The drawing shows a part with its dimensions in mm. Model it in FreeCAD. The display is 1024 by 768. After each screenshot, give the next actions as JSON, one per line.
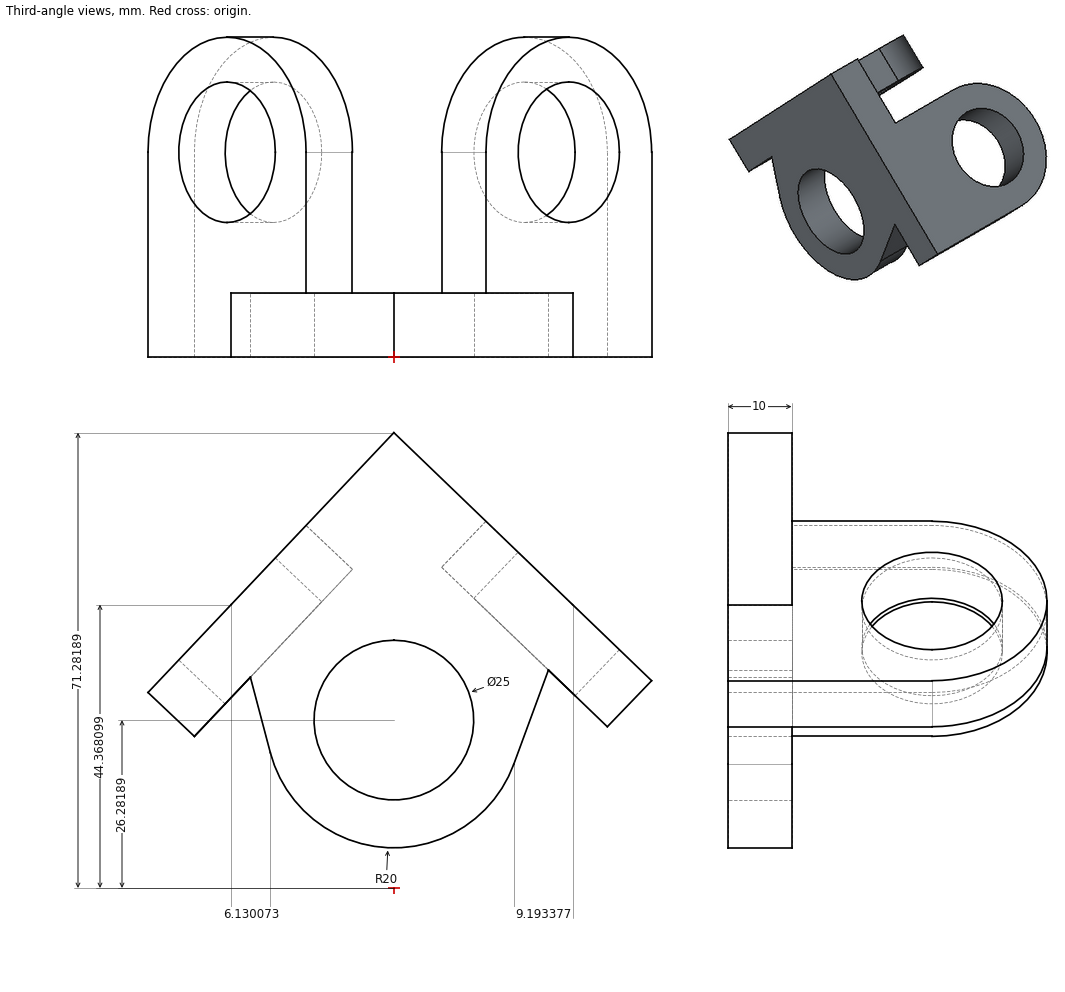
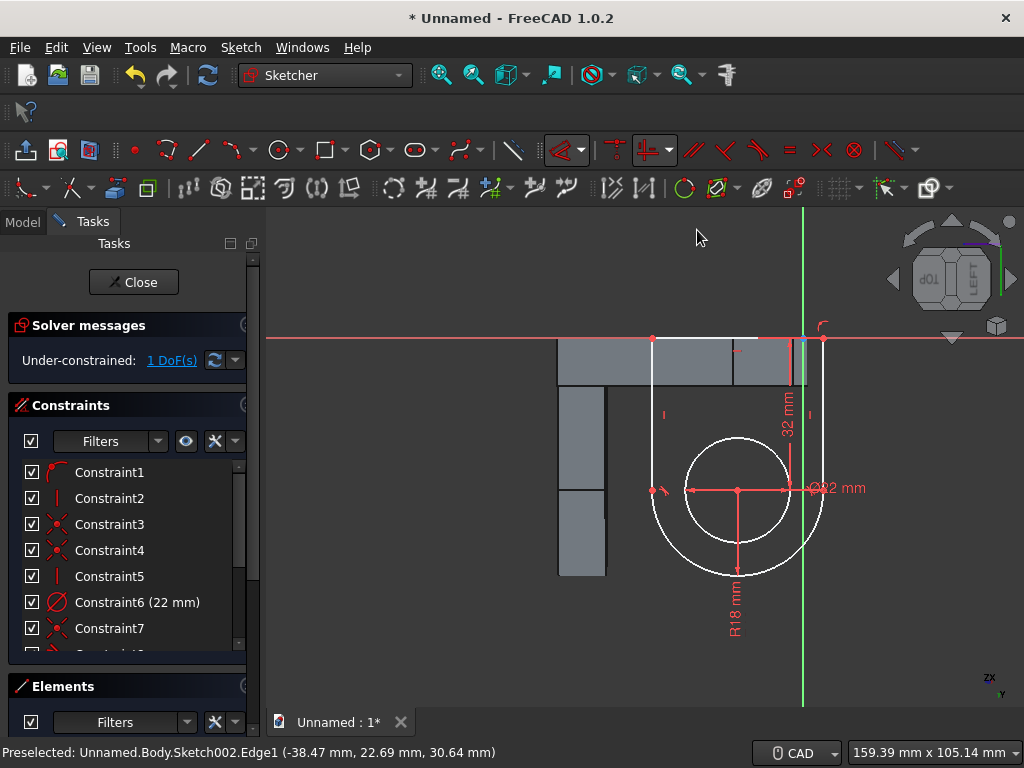
{"action": "scroll", "coordinate": [823, 490], "scroll_direction": "up", "scroll_amount": 4}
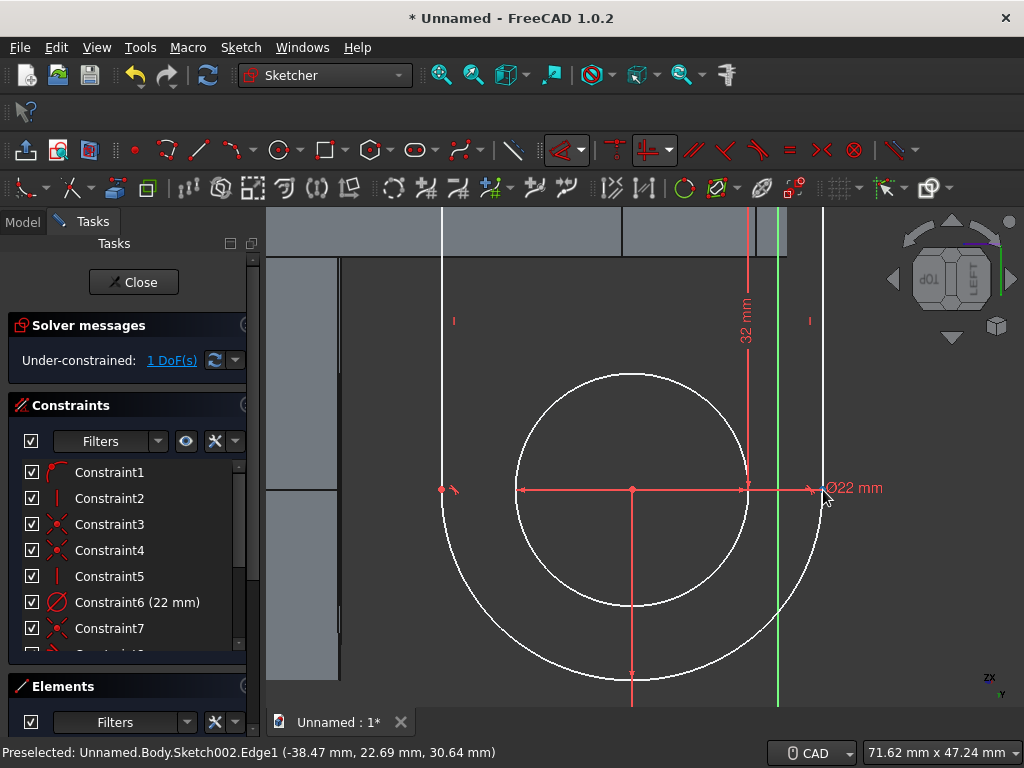
{"action": "left_click", "coordinate": [823, 490]}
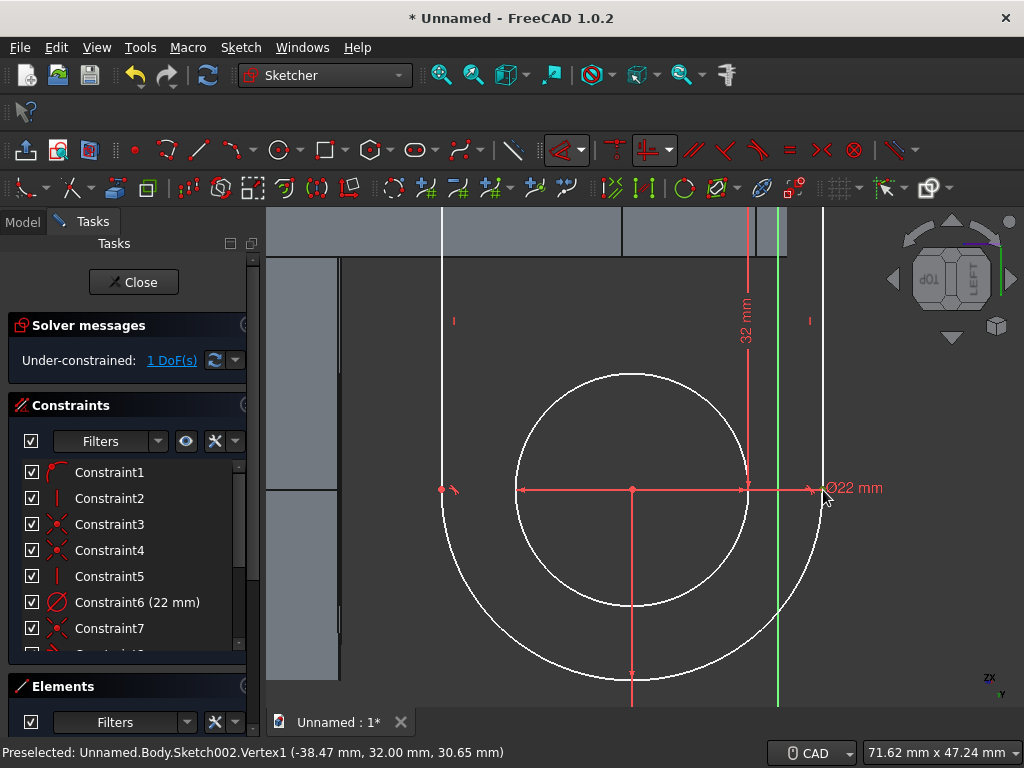
{"action": "key", "text": "l"}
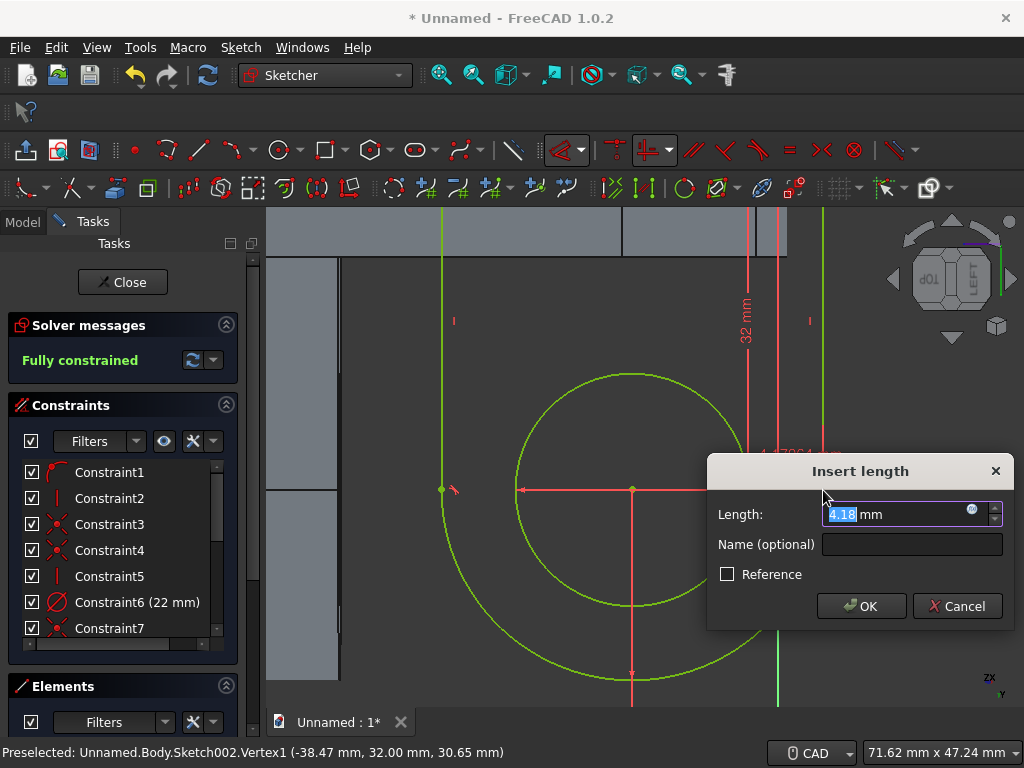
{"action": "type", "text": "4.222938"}
{"action": "key", "text": "Return"}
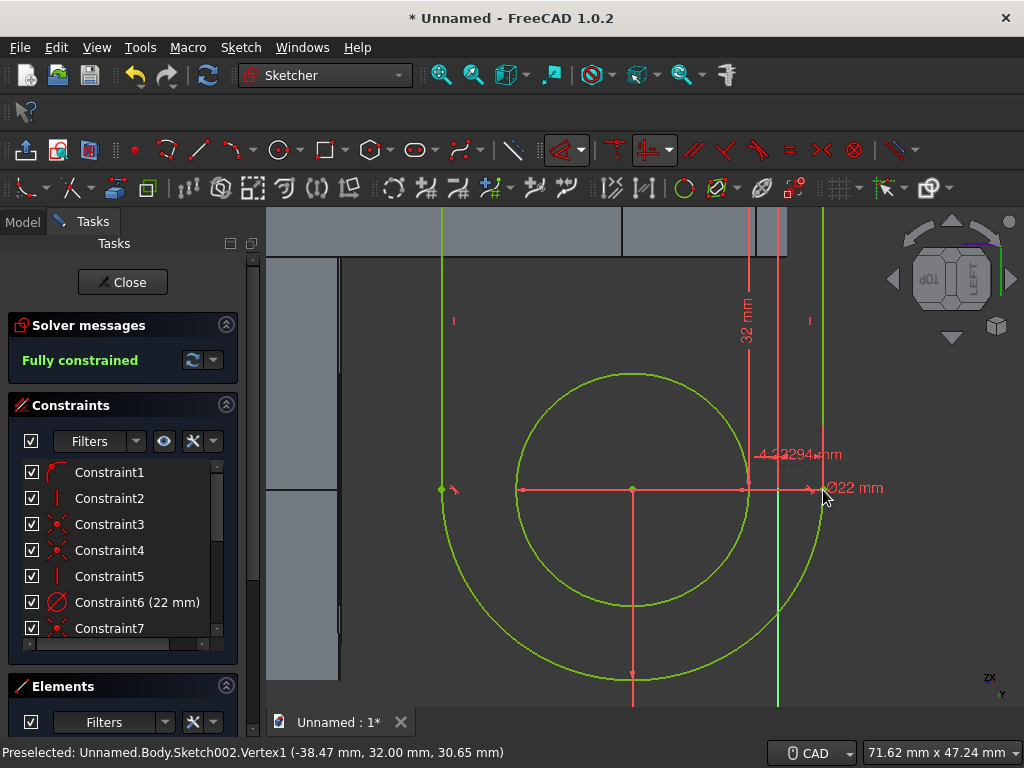
{"action": "left_click", "coordinate": [123, 282]}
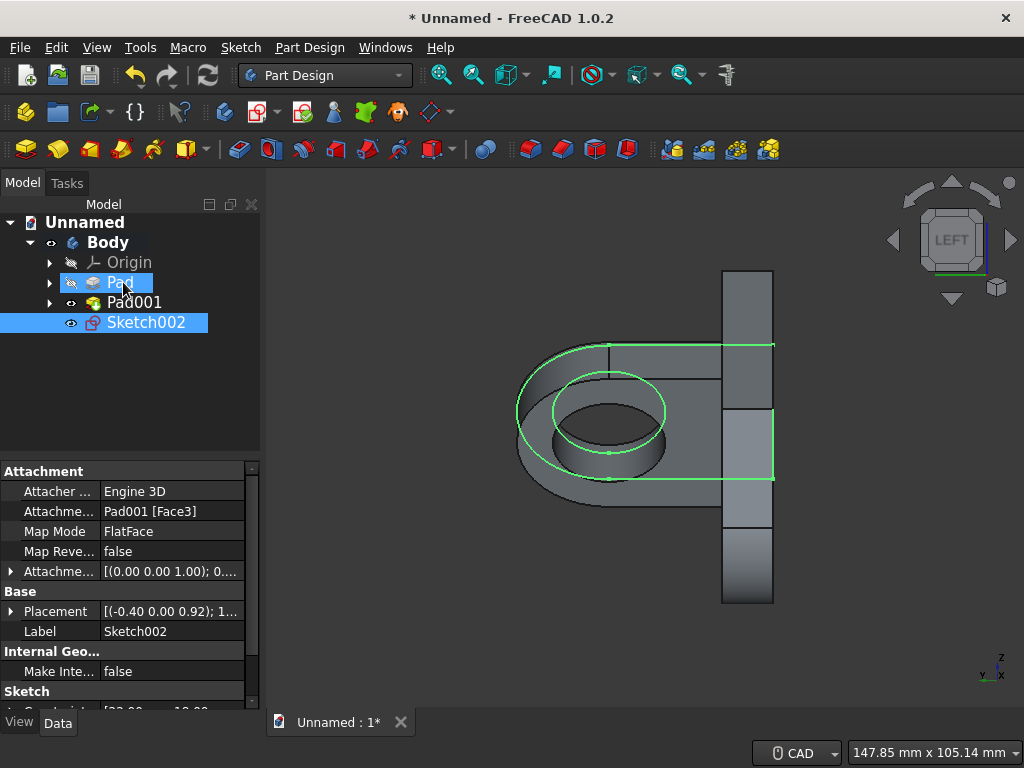
{"action": "left_click", "coordinate": [26, 150]}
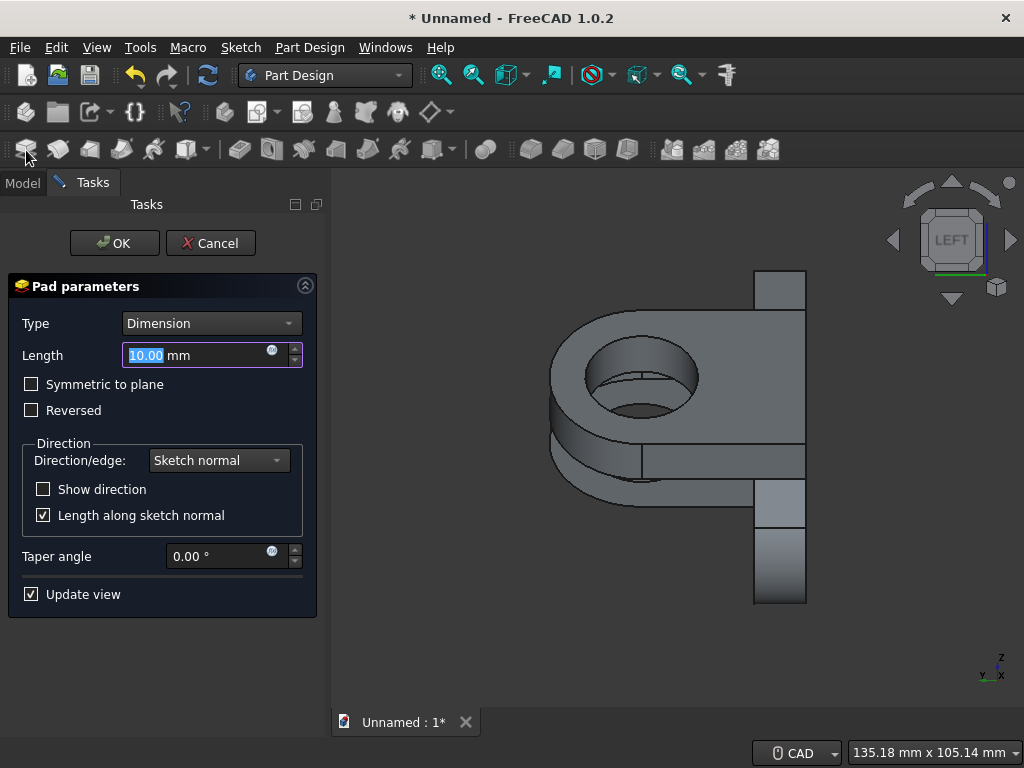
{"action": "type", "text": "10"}
{"action": "key", "text": "Tab"}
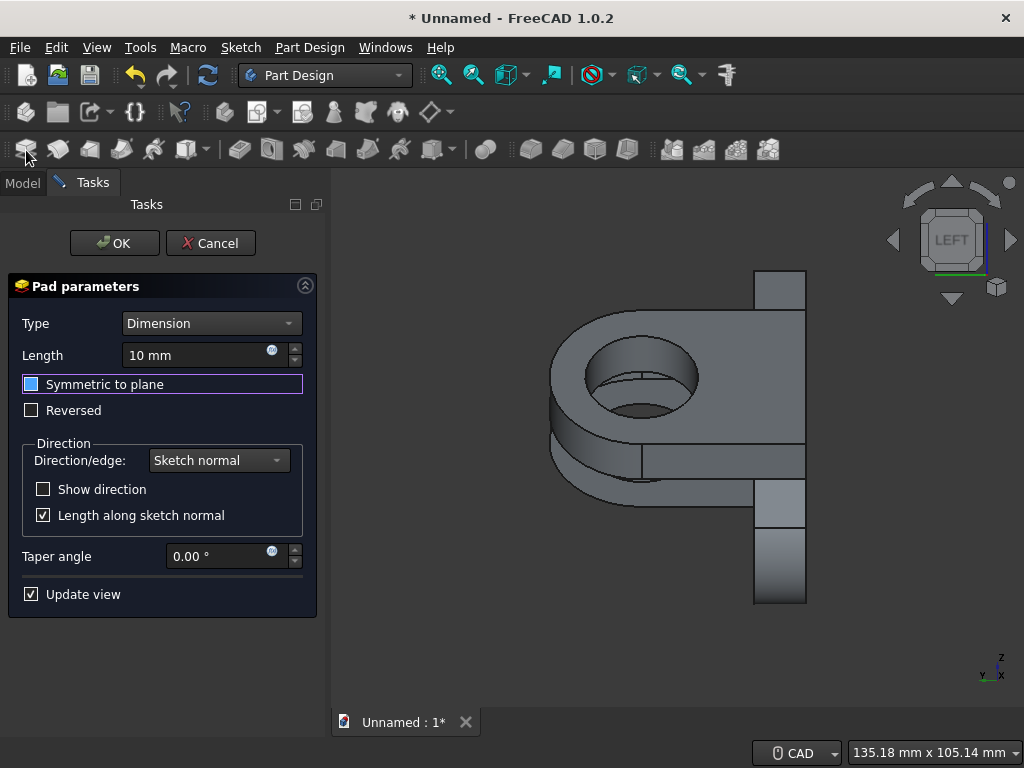
{"action": "left_click", "coordinate": [30, 410]}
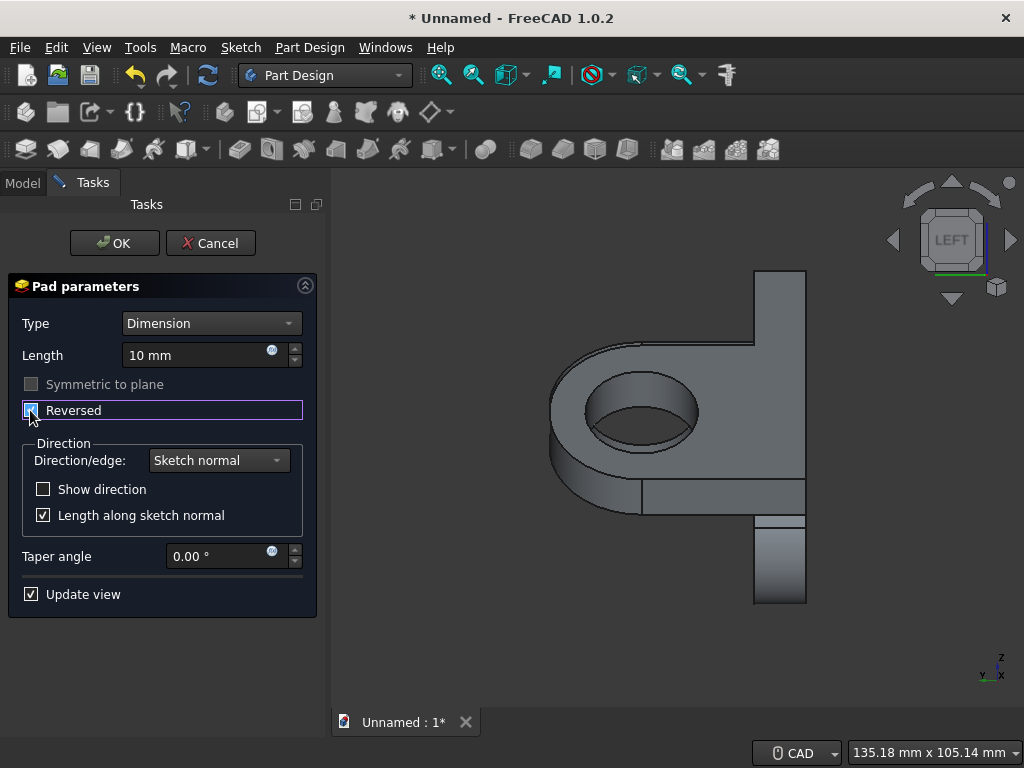
{"action": "left_click", "coordinate": [115, 243]}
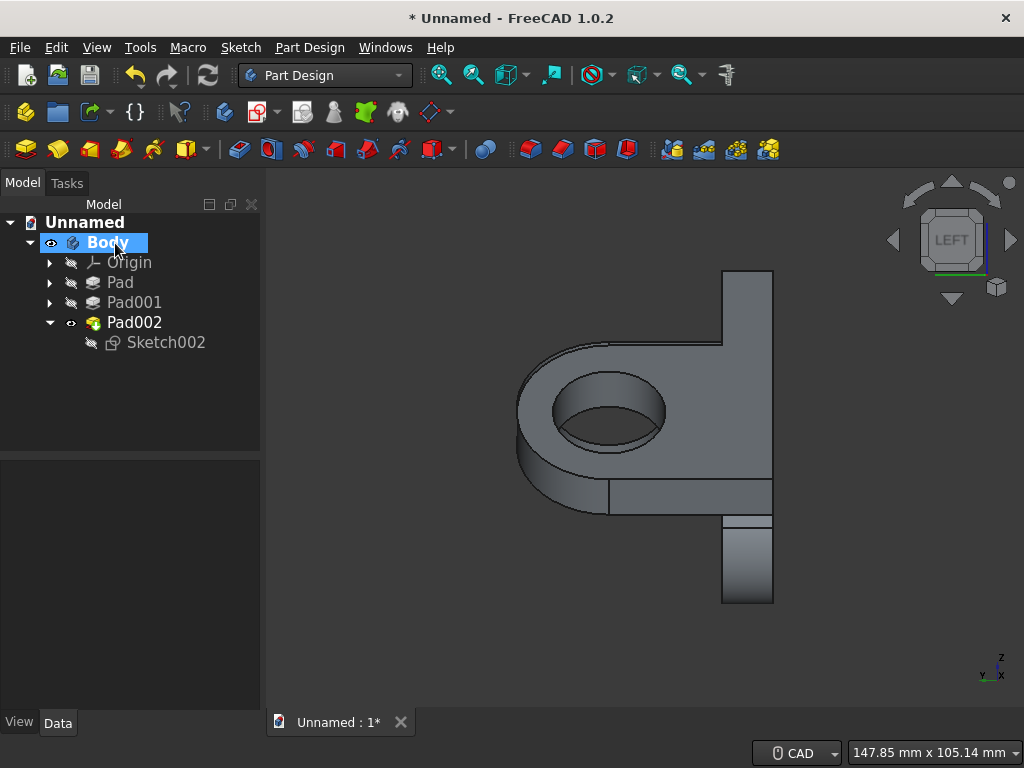
{"action": "key", "text": "0"}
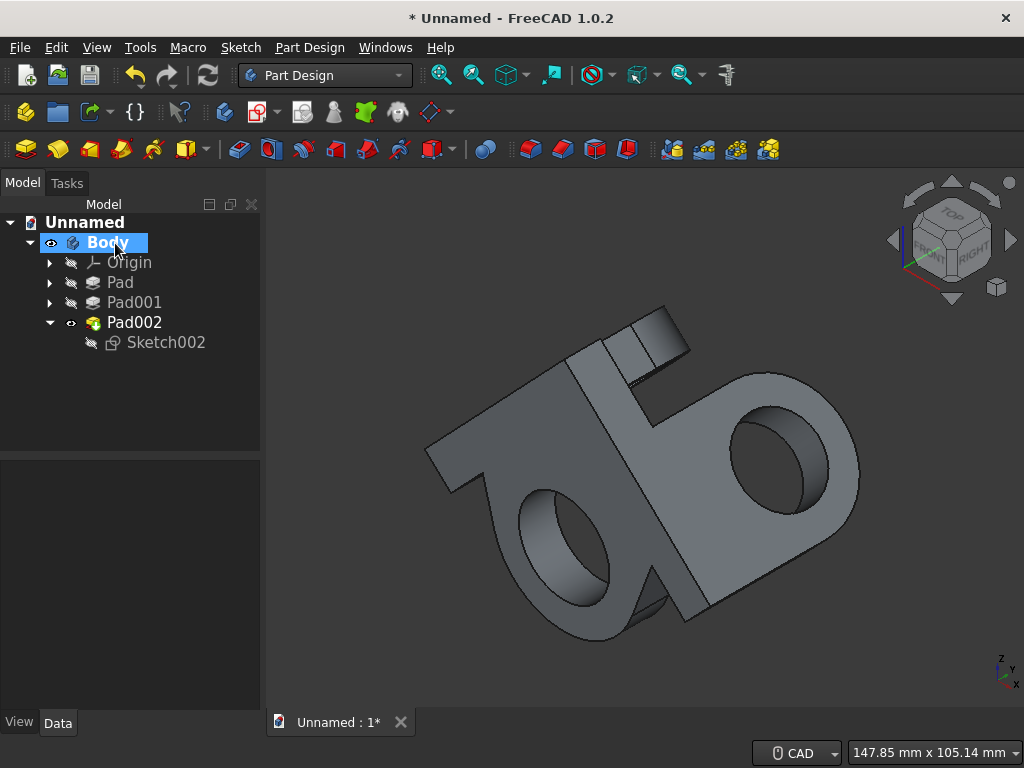
{"action": "left_click", "coordinate": [442, 76]}